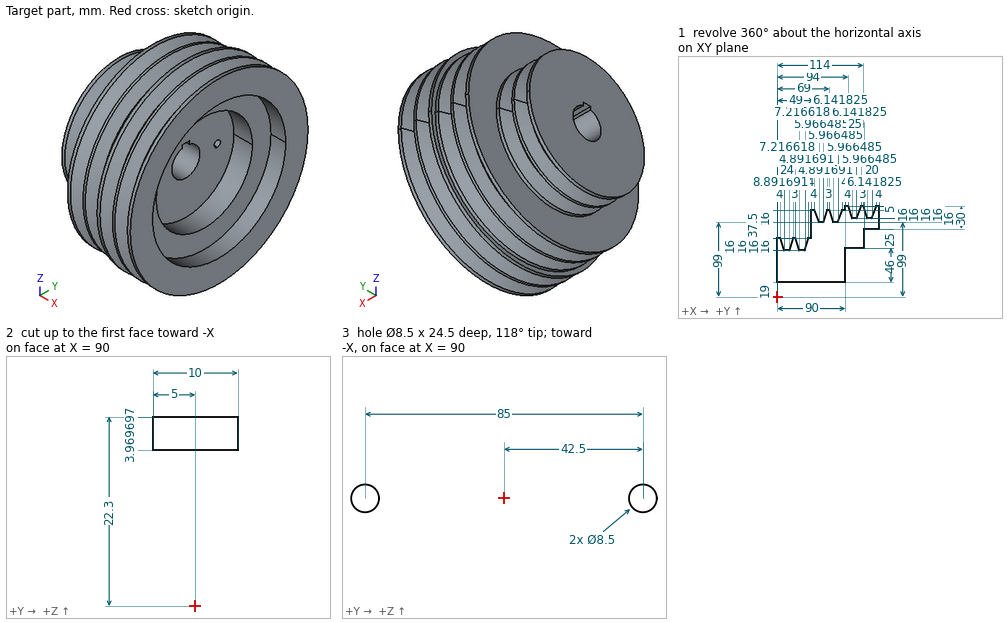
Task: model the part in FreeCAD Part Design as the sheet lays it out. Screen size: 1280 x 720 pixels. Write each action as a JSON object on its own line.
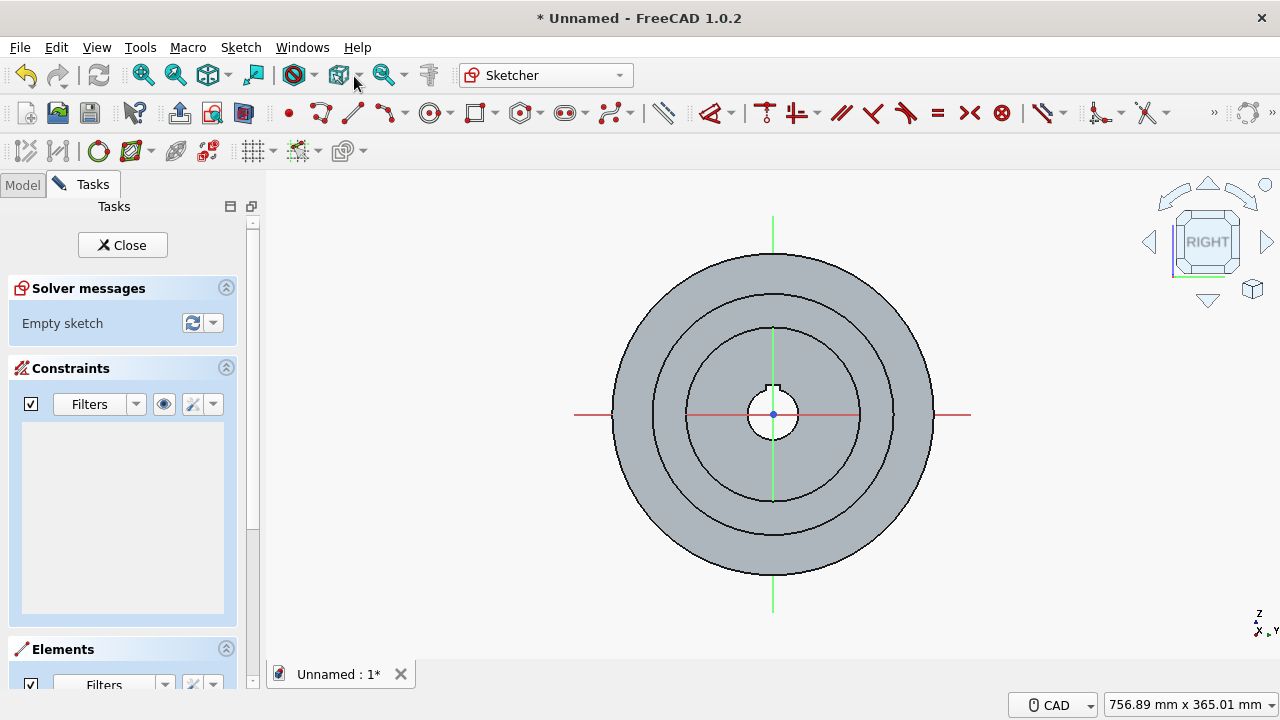
{"action": "scroll", "coordinate": [790, 414], "scroll_direction": "up", "scroll_amount": 8}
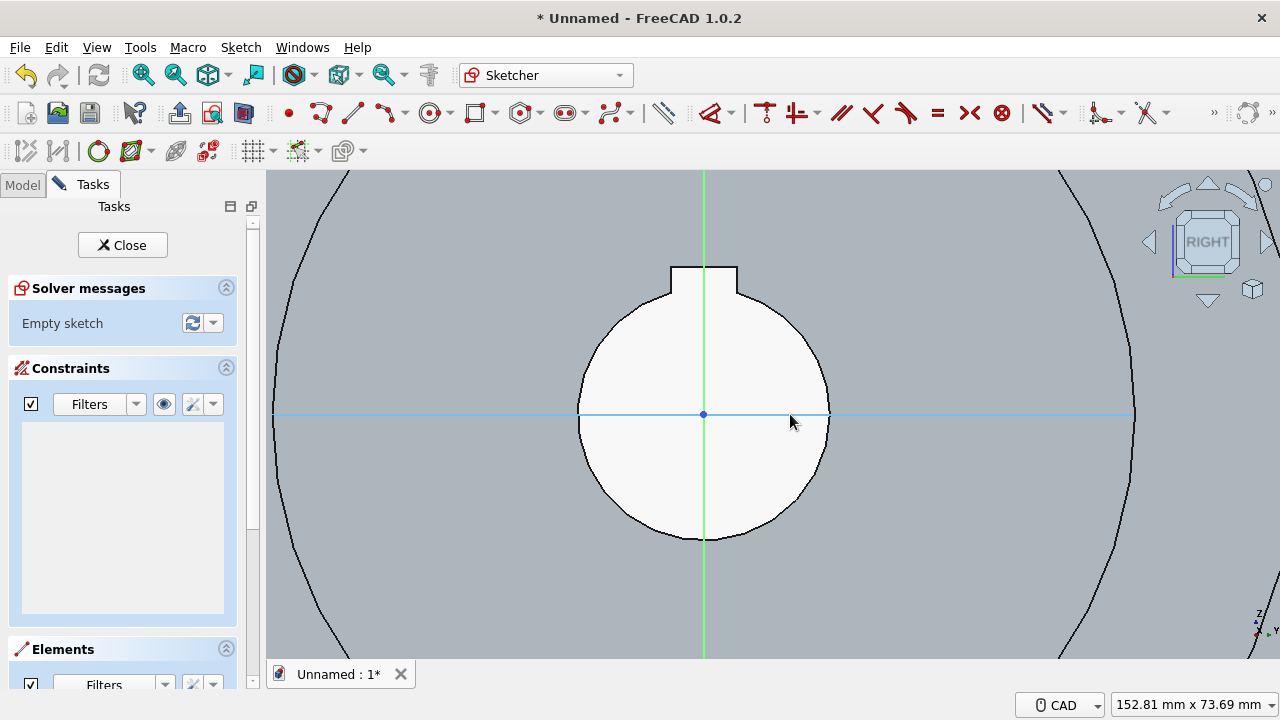
{"action": "key", "text": "g c"}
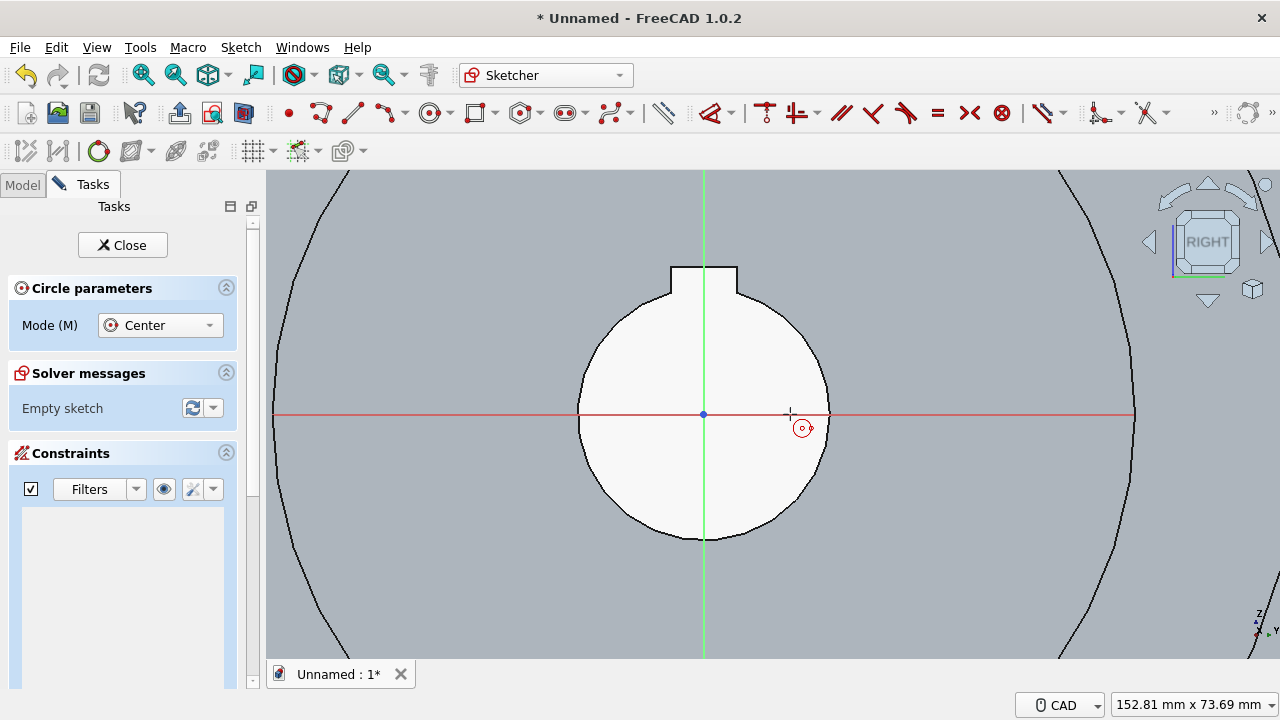
{"action": "left_click", "coordinate": [986, 414]}
{"action": "left_click", "coordinate": [1006, 395]}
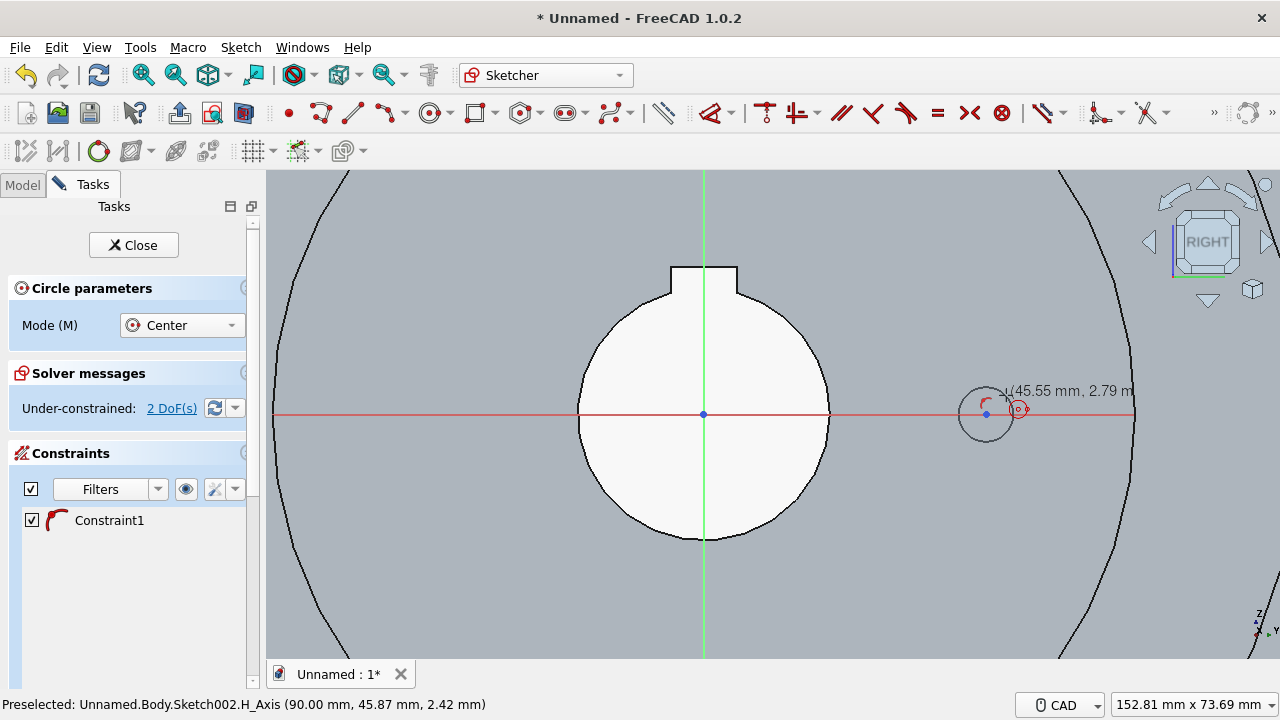
{"action": "left_click", "coordinate": [422, 414]}
{"action": "left_click", "coordinate": [442, 395]}
{"action": "key", "text": "Escape"}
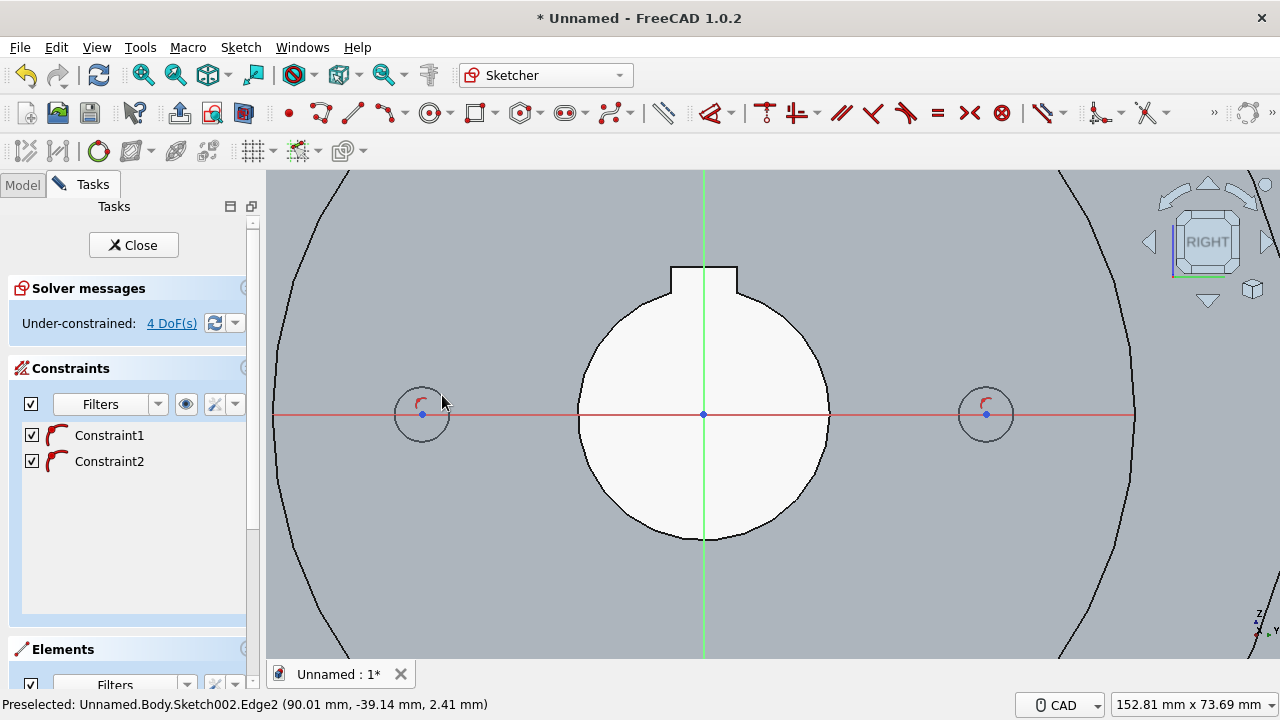
{"action": "left_click", "coordinate": [1005, 395]}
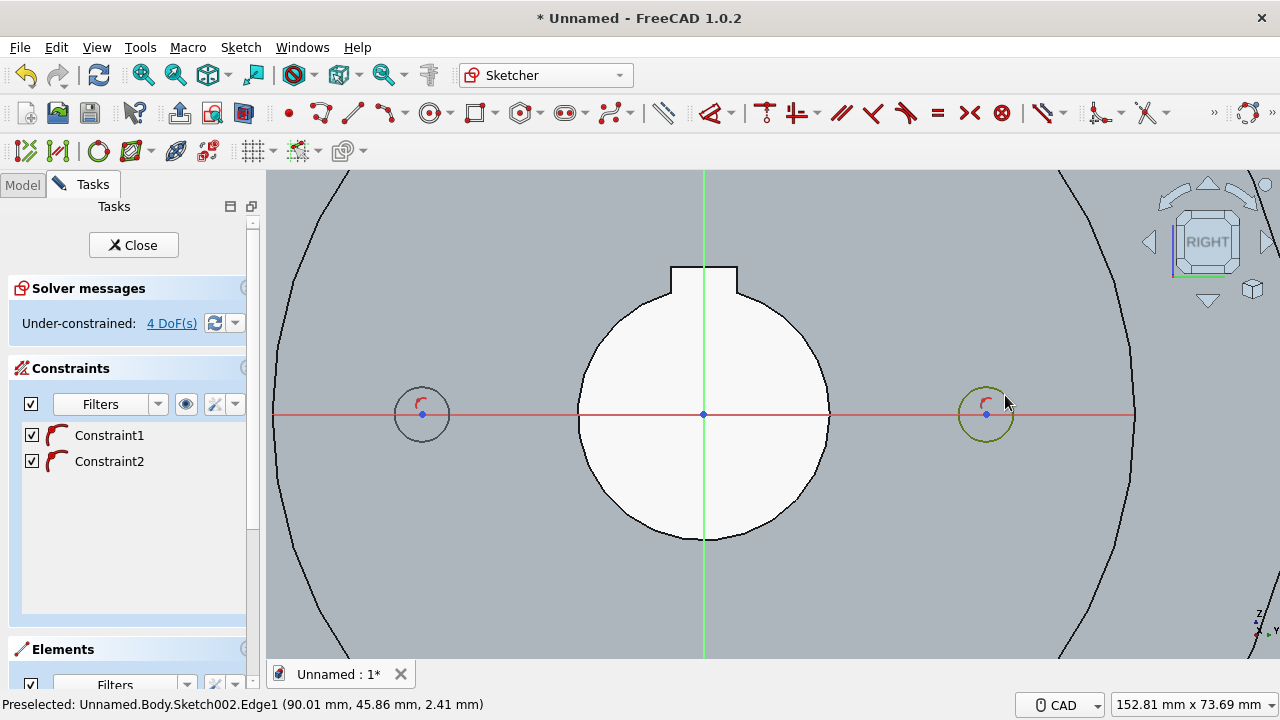
{"action": "left_click", "coordinate": [441, 395]}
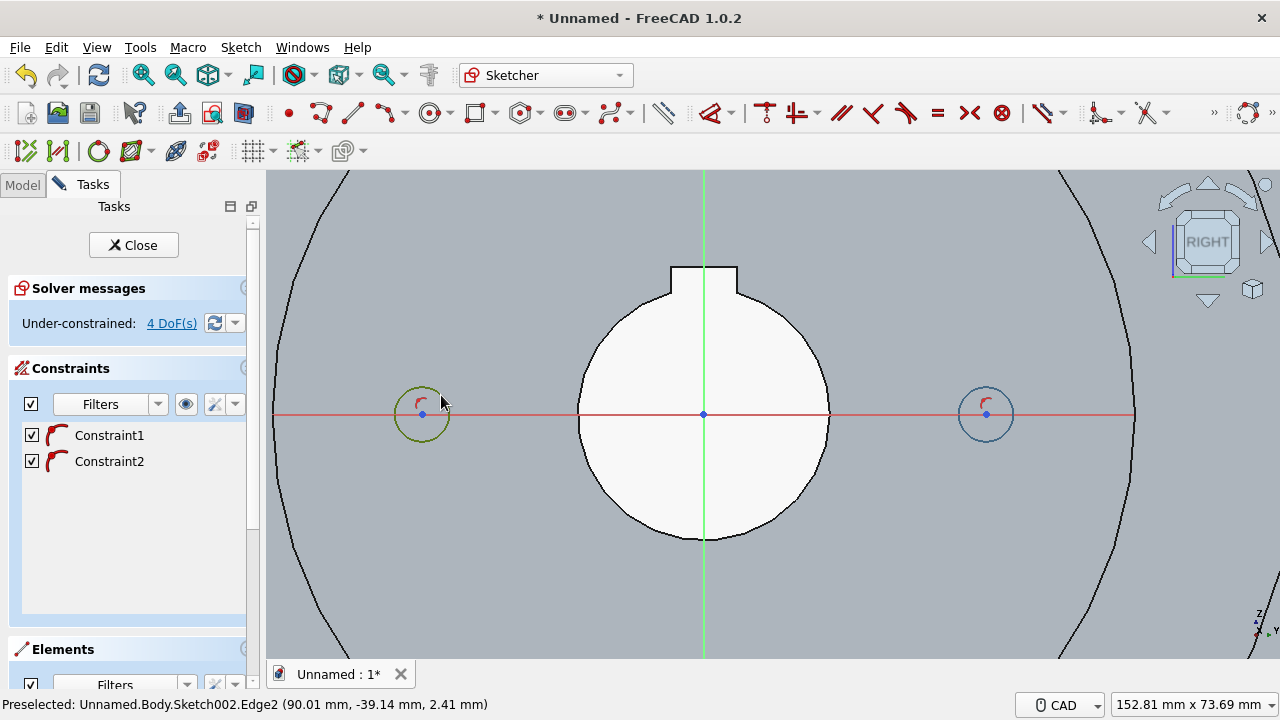
{"action": "key", "text": "e"}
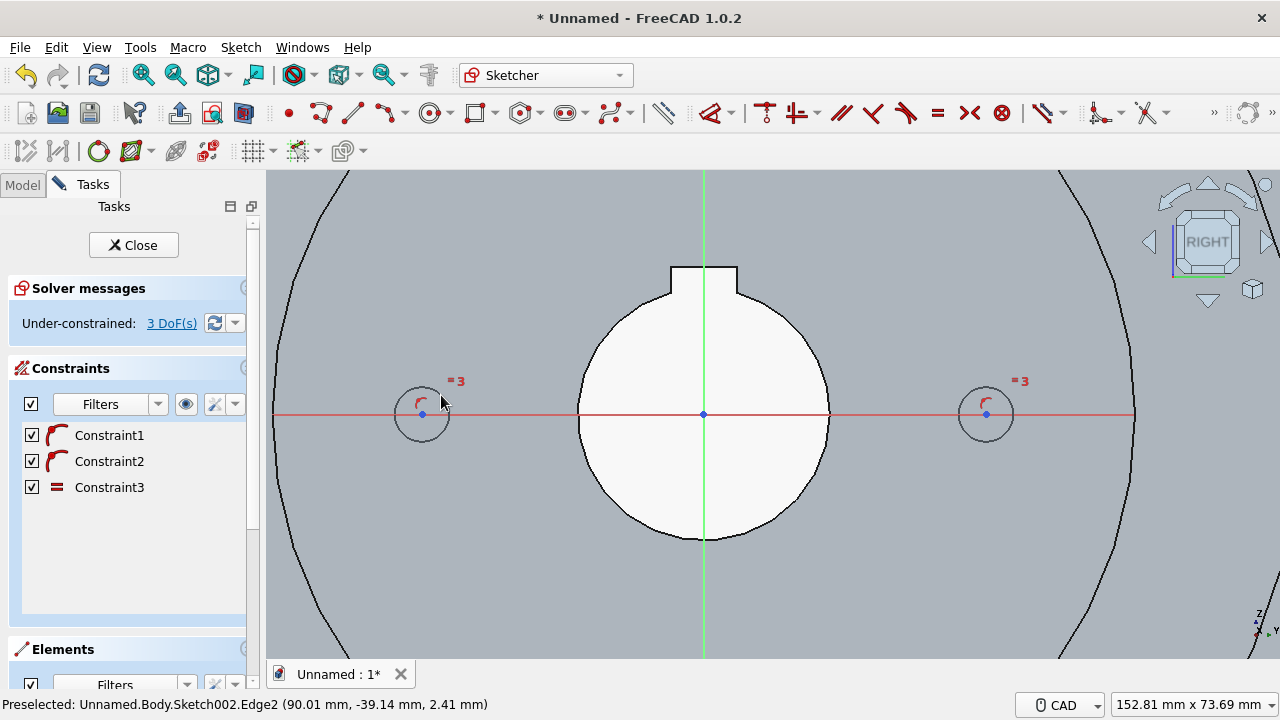
{"action": "key", "text": "d"}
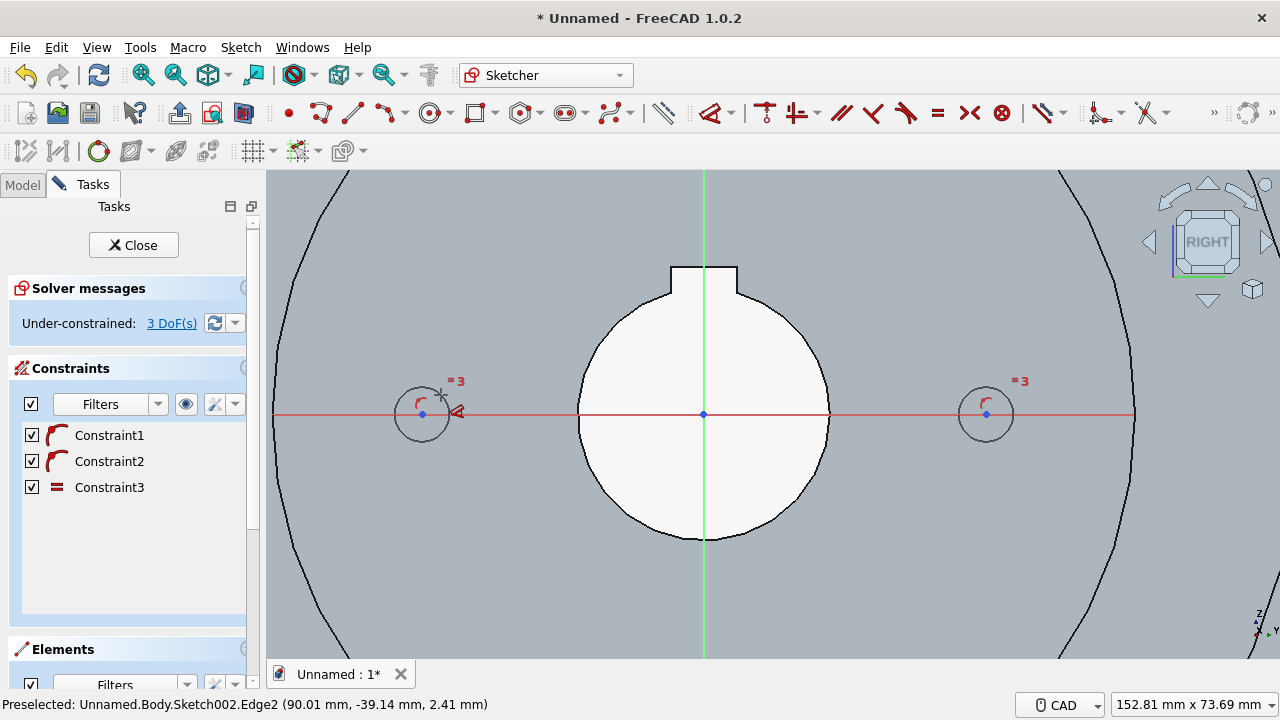
{"action": "left_click", "coordinate": [1005, 395]}
{"action": "left_click", "coordinate": [1027, 372]}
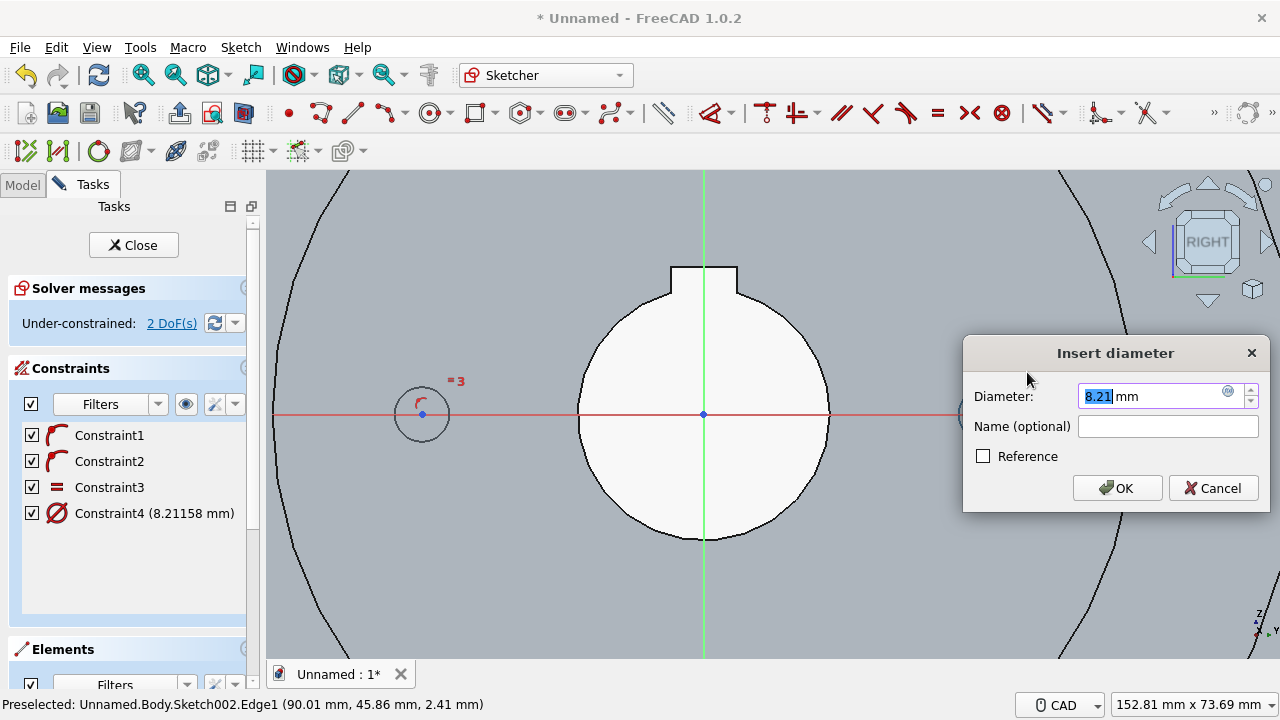
{"action": "type", "text": "8.5"}
{"action": "key", "text": "Return"}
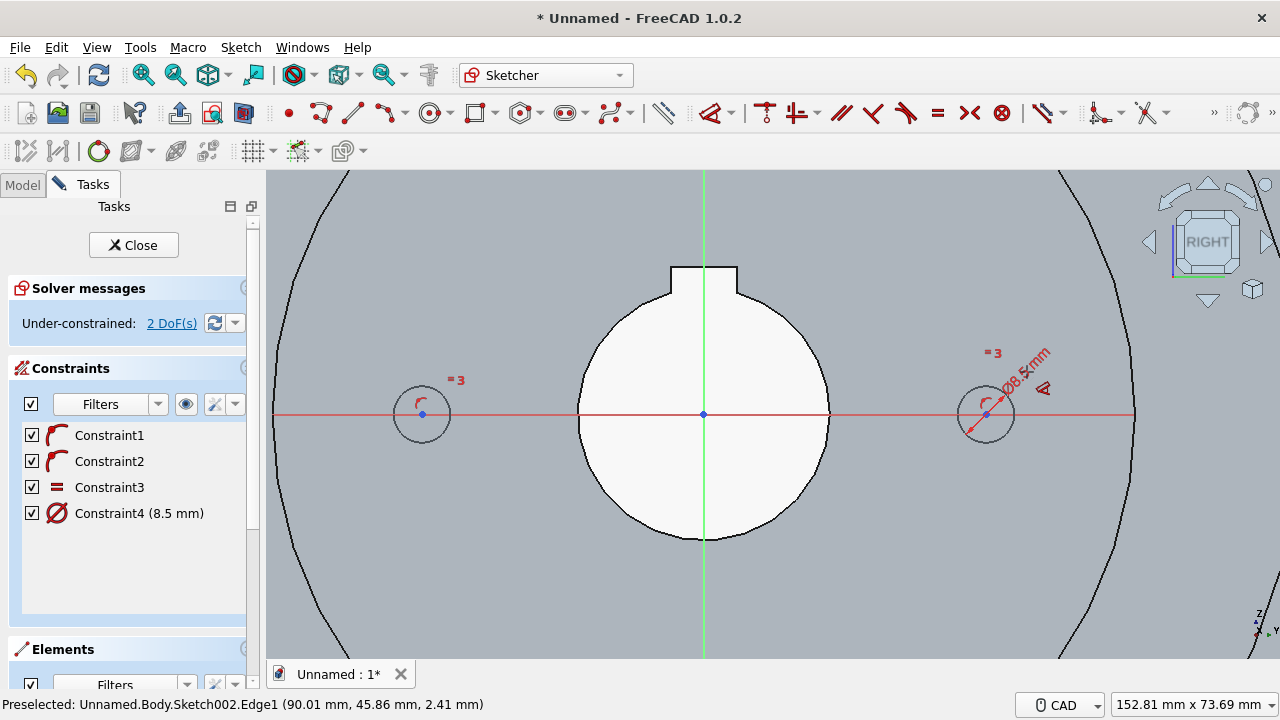
{"action": "left_click", "coordinate": [986, 414]}